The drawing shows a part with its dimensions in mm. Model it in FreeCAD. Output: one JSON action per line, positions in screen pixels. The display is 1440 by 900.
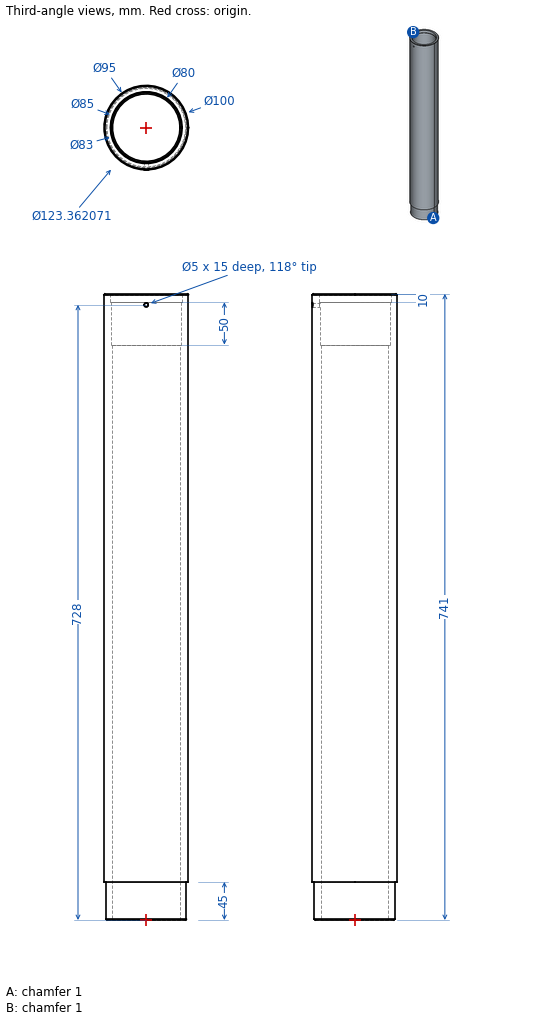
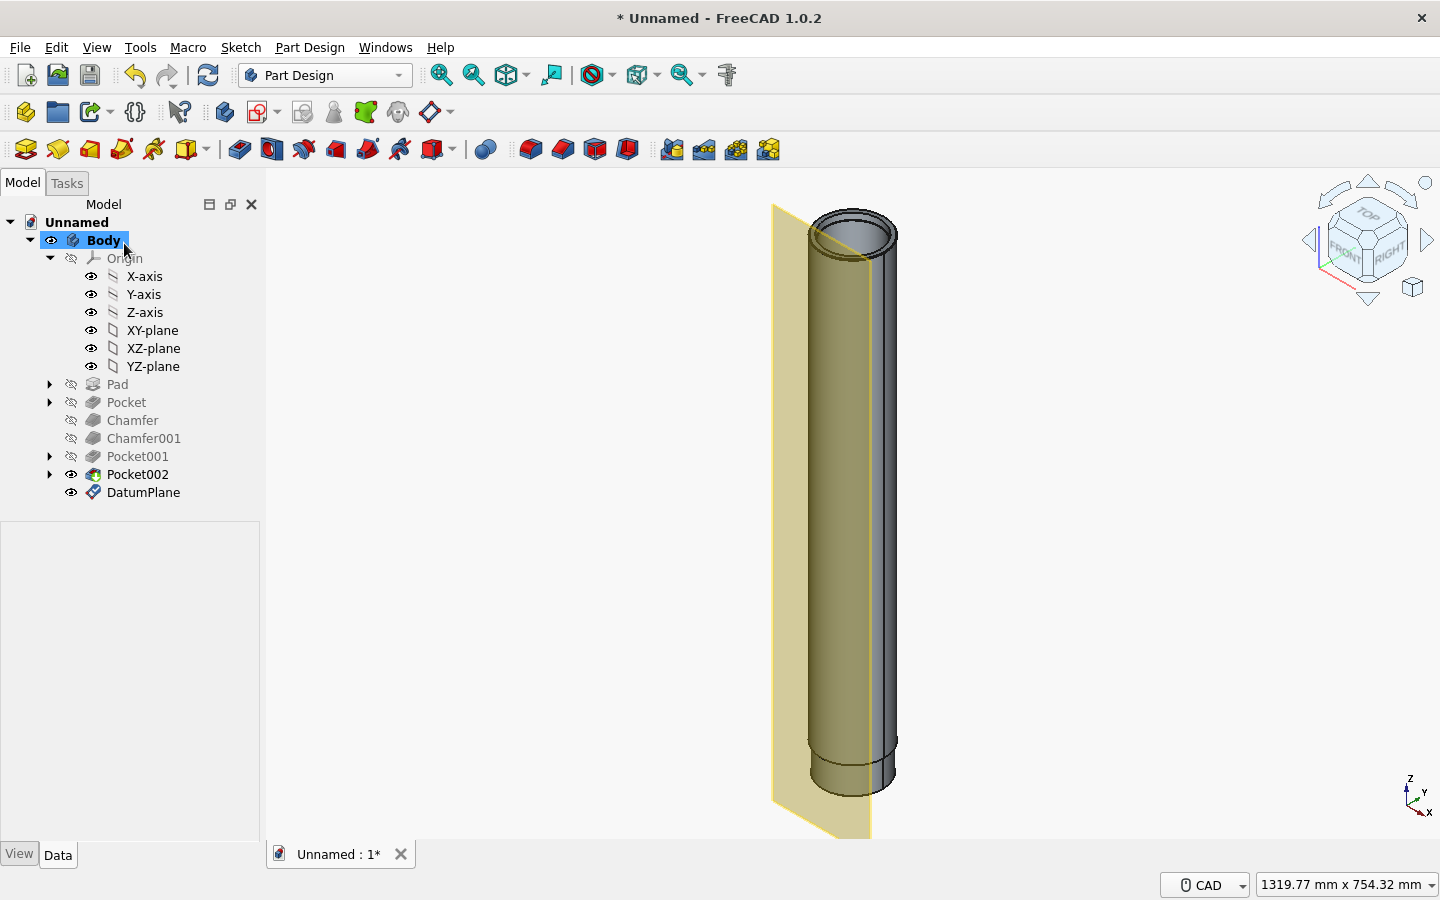
{"action": "left_click", "coordinate": [116, 492]}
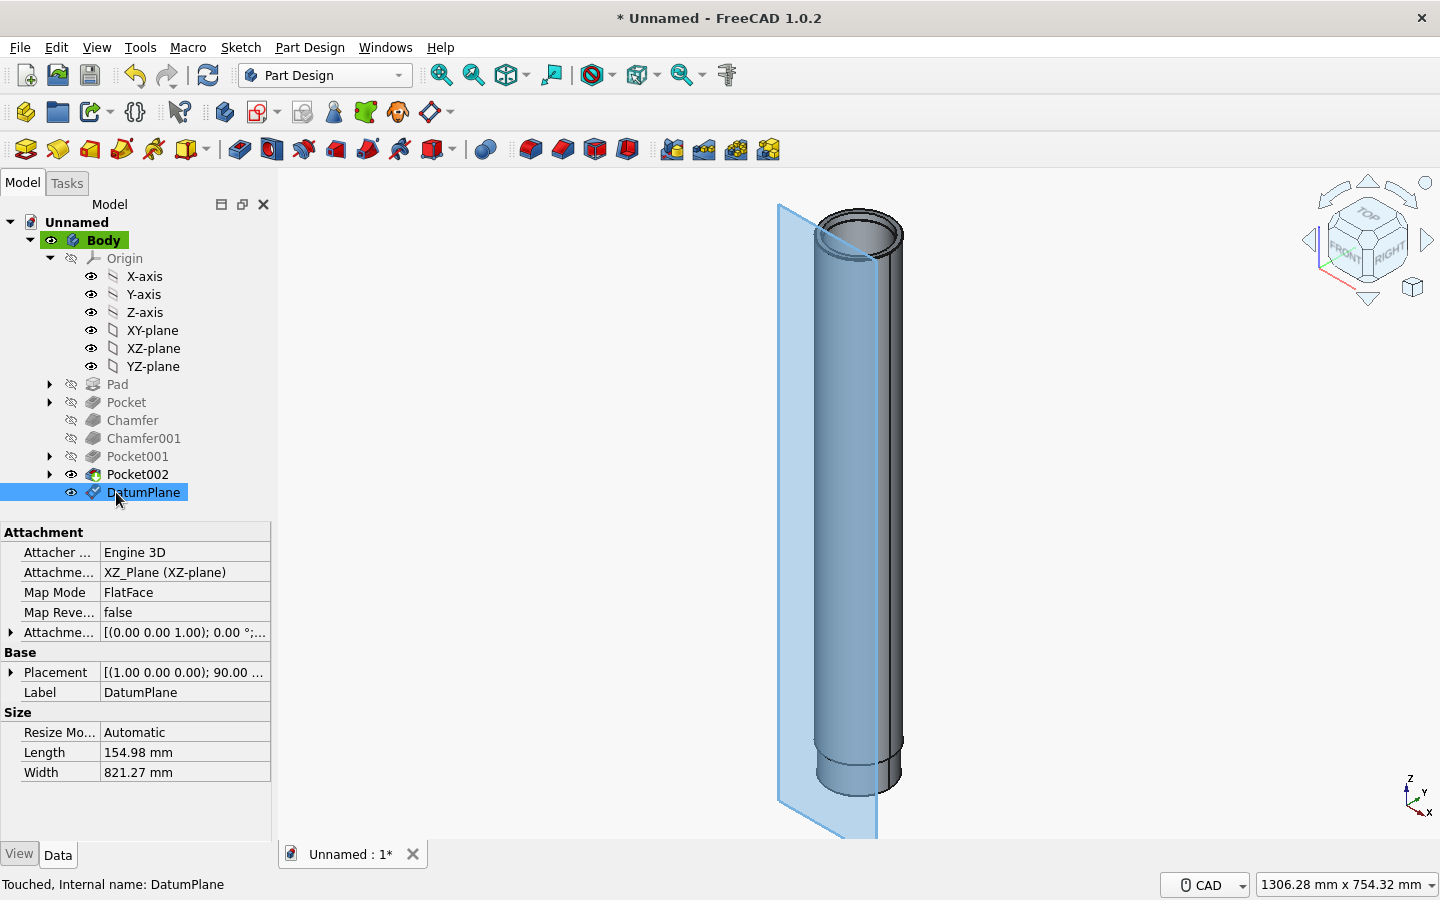
{"action": "left_click", "coordinate": [258, 112]}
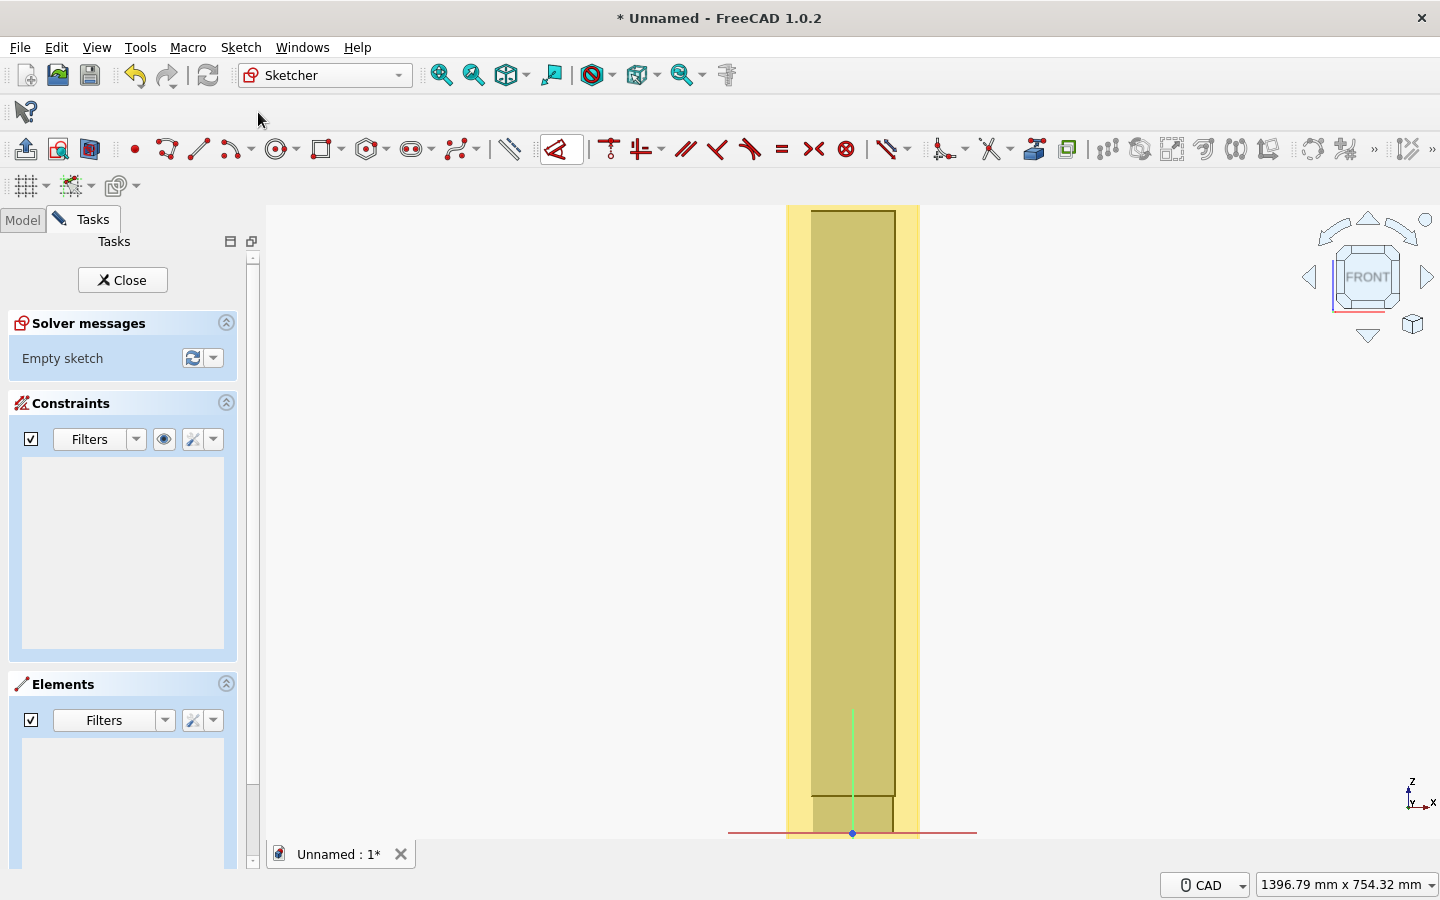
{"action": "scroll", "coordinate": [784, 522], "scroll_direction": "down", "scroll_amount": 5}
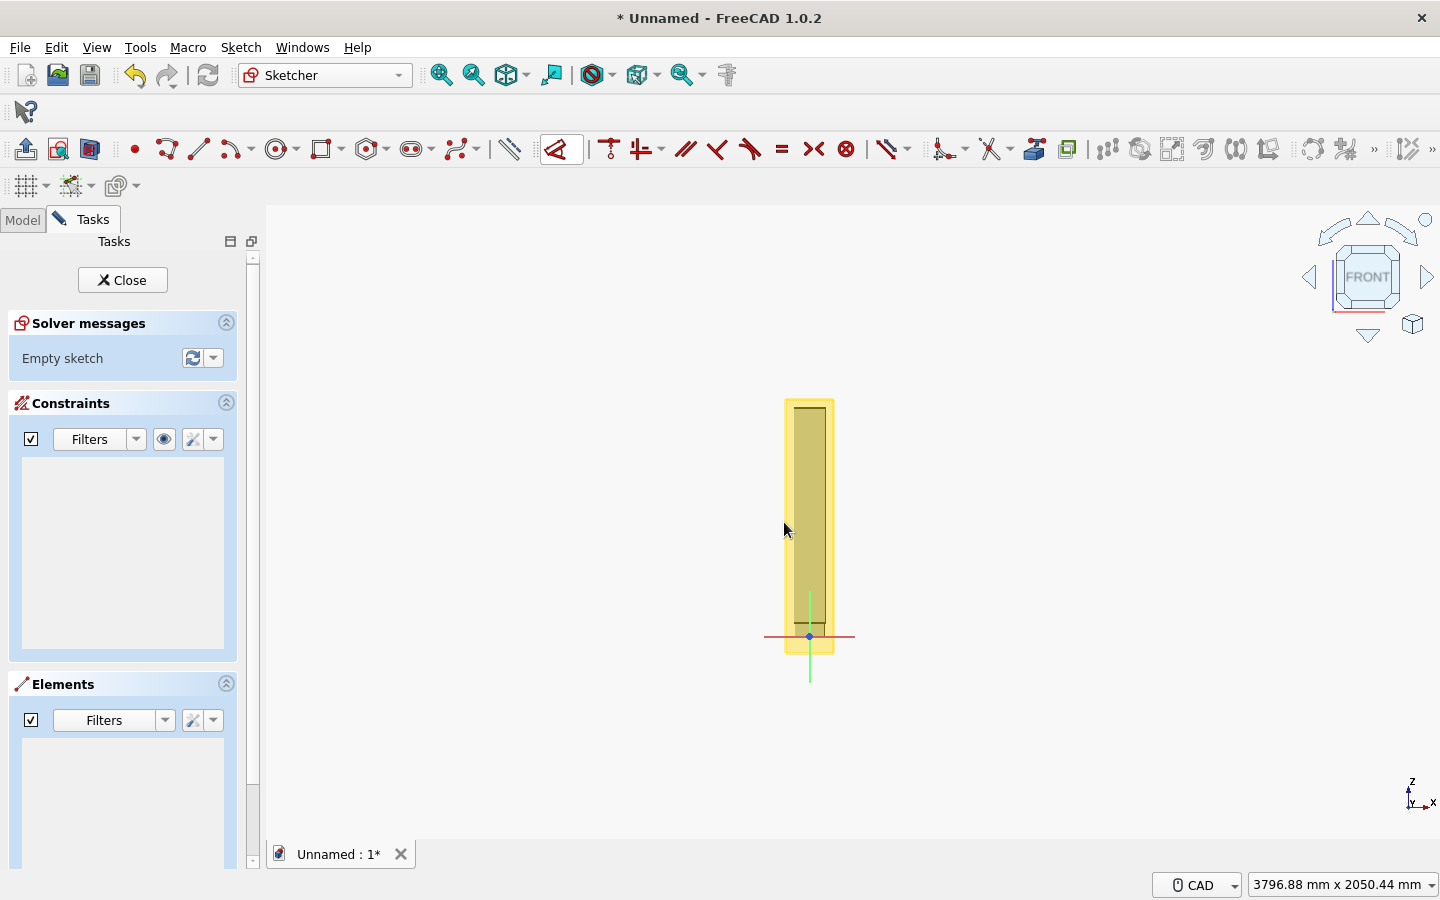
{"action": "scroll", "coordinate": [811, 406], "scroll_direction": "up", "scroll_amount": 15}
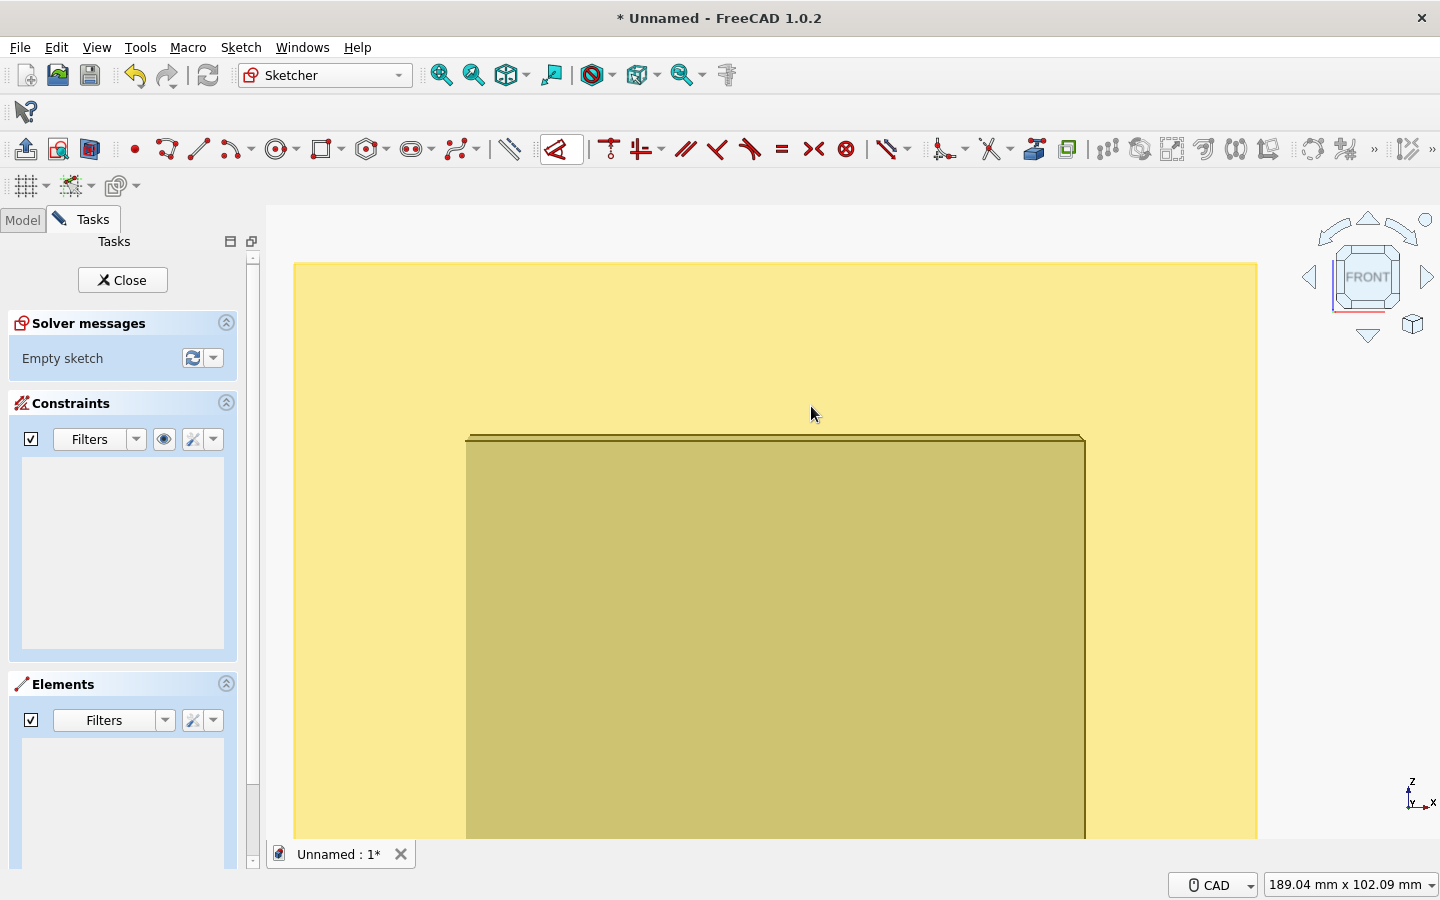
{"action": "scroll", "coordinate": [774, 515], "scroll_direction": "up", "scroll_amount": 13}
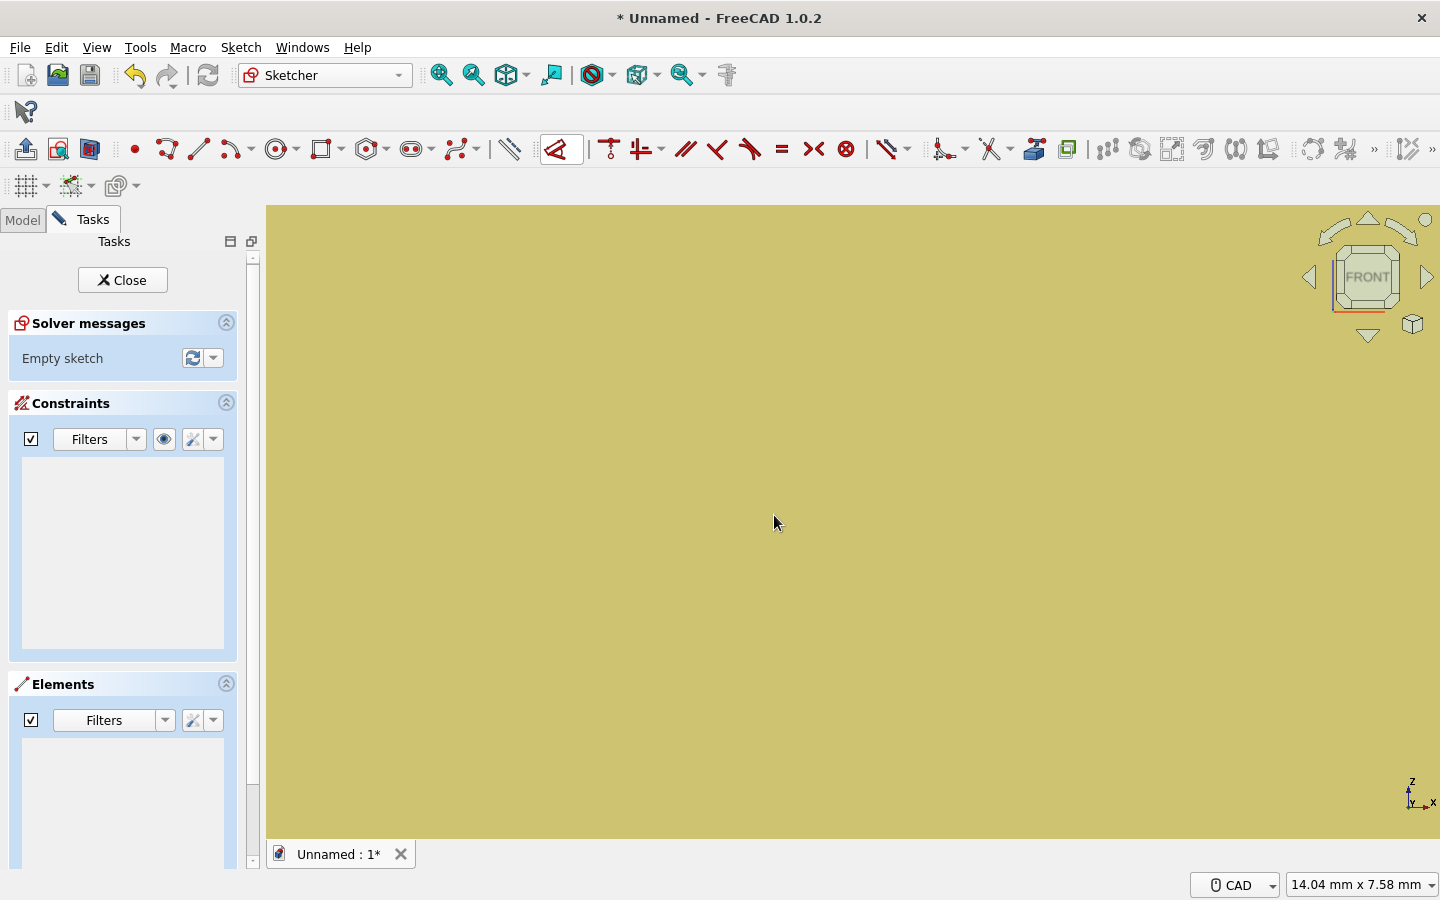
{"action": "left_click", "coordinate": [276, 150]}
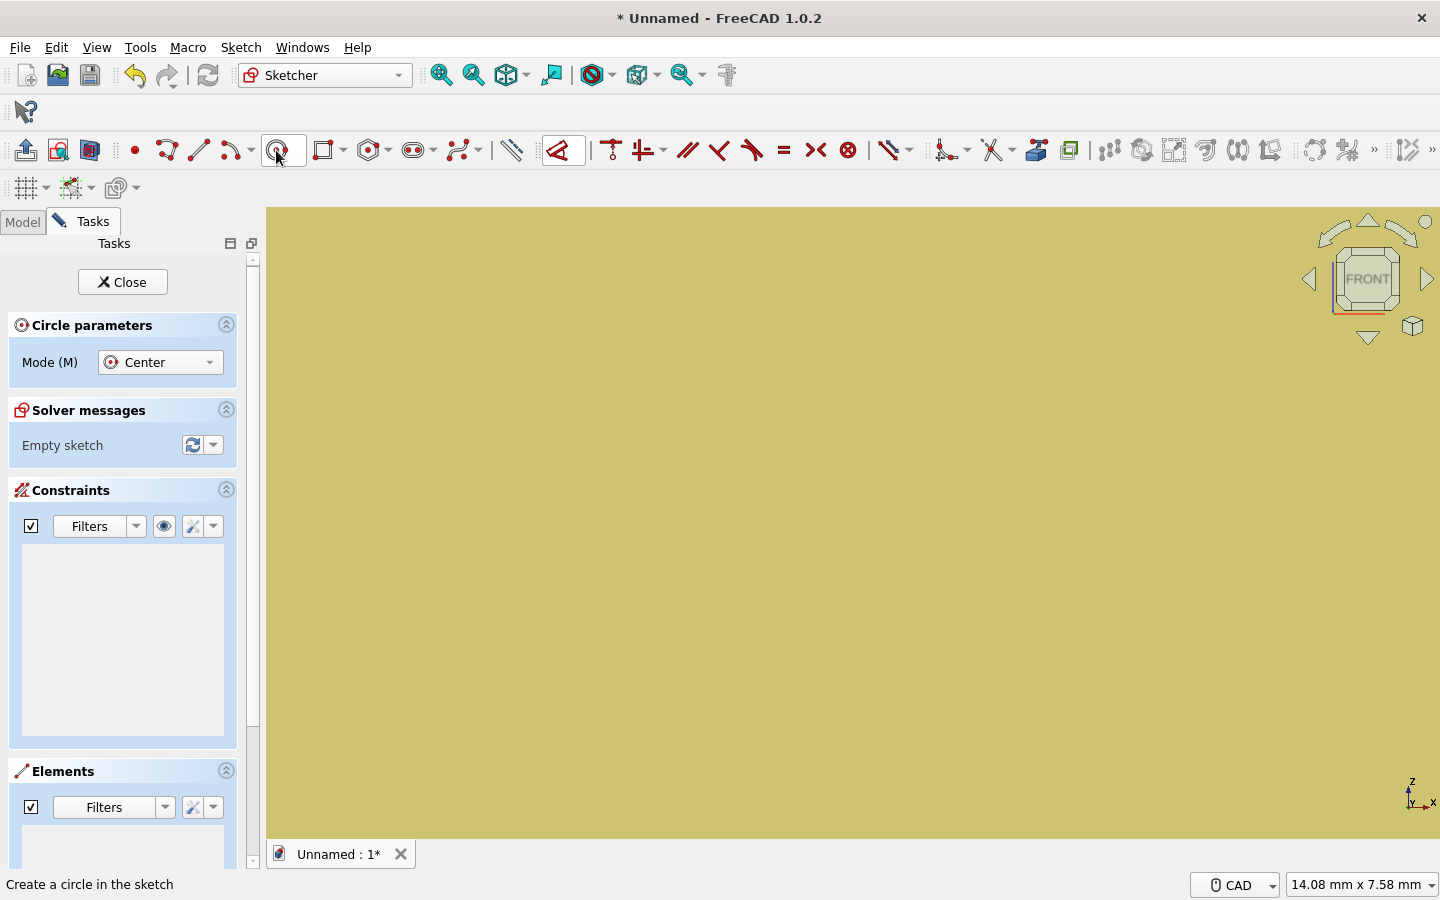
{"action": "left_click", "coordinate": [774, 523]}
{"action": "left_click", "coordinate": [921, 376]}
{"action": "key", "text": "Escape"}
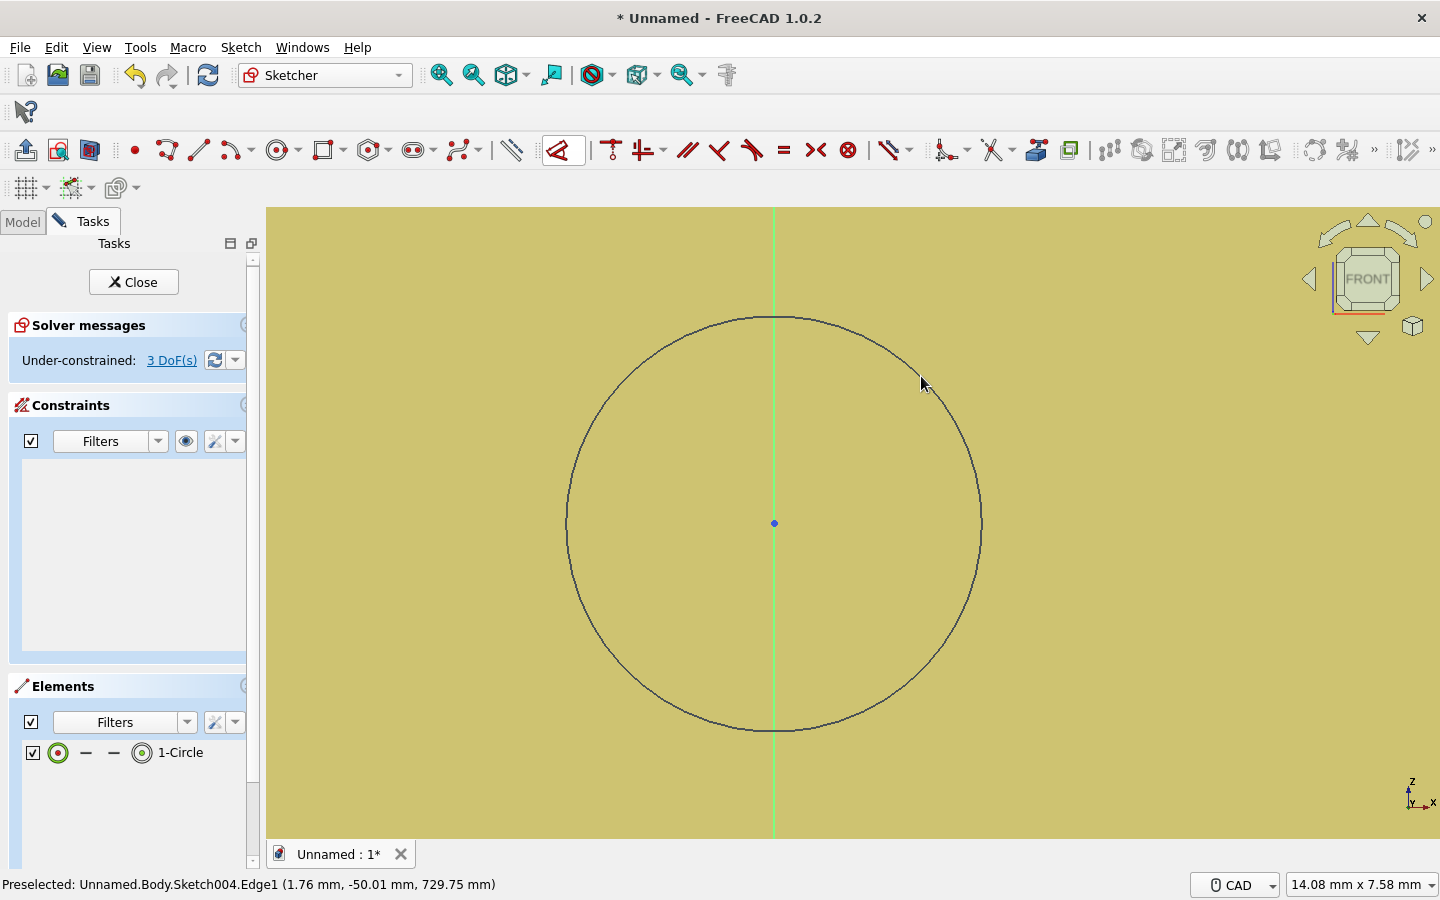
{"action": "left_click", "coordinate": [774, 524]}